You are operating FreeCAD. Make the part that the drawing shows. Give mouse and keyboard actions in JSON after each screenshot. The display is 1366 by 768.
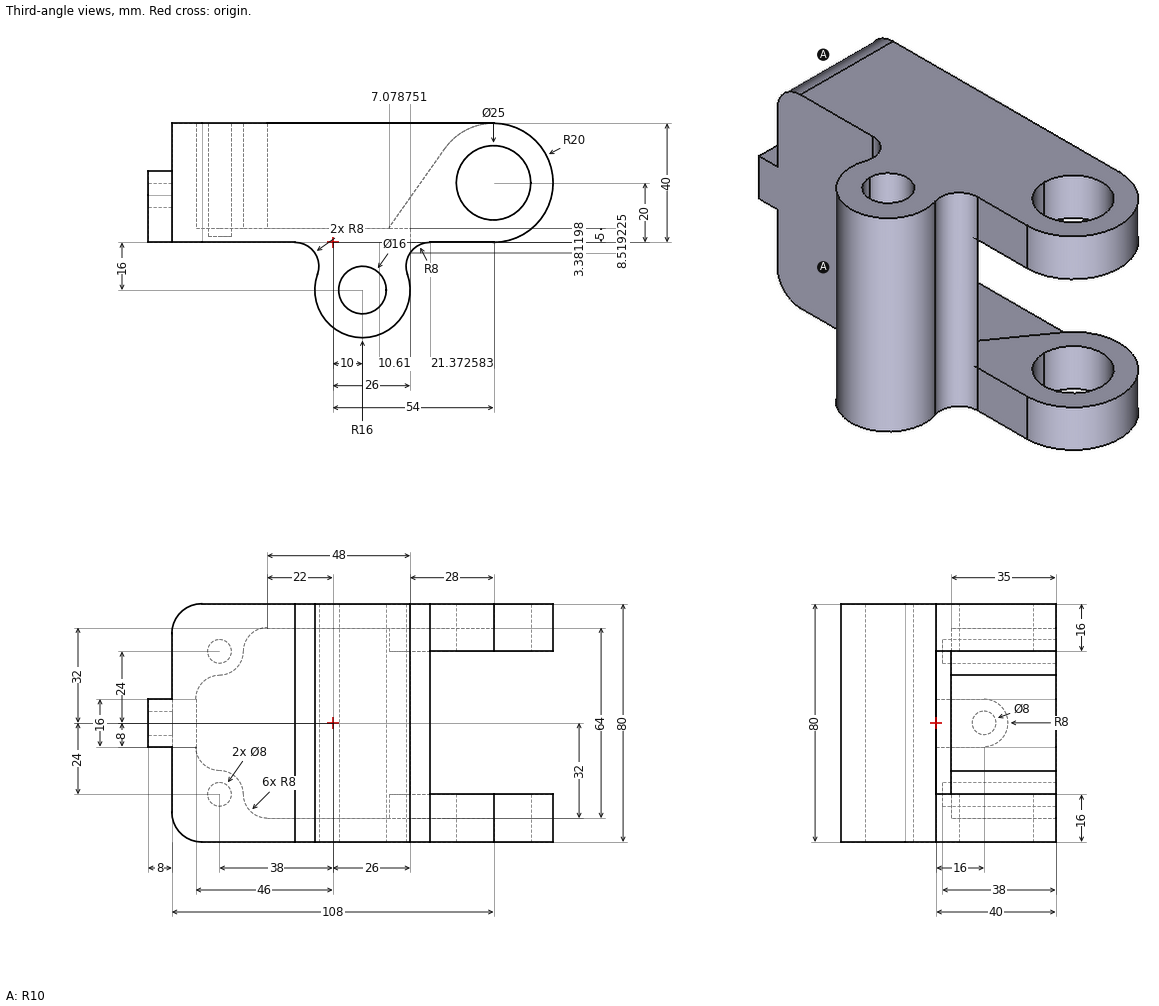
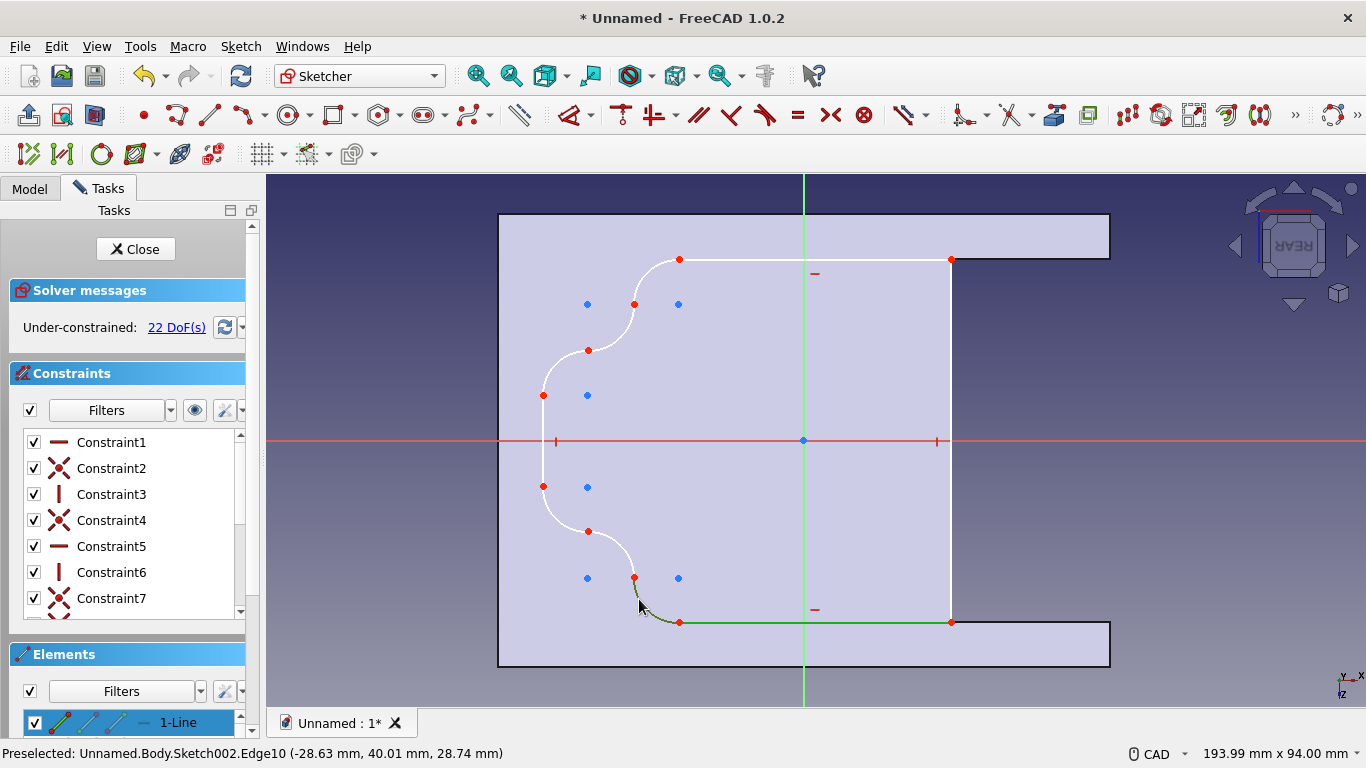
{"action": "key", "text": "t"}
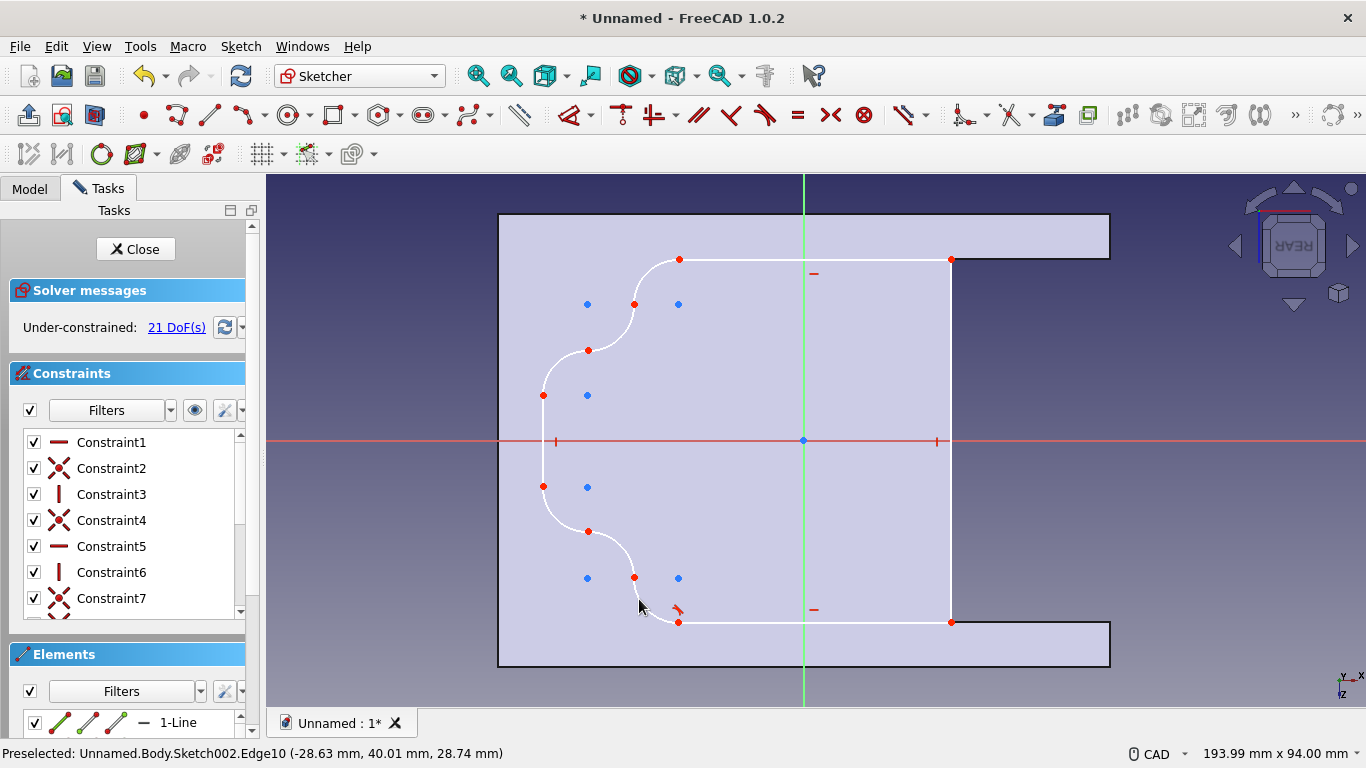
{"action": "left_click", "coordinate": [869, 260]}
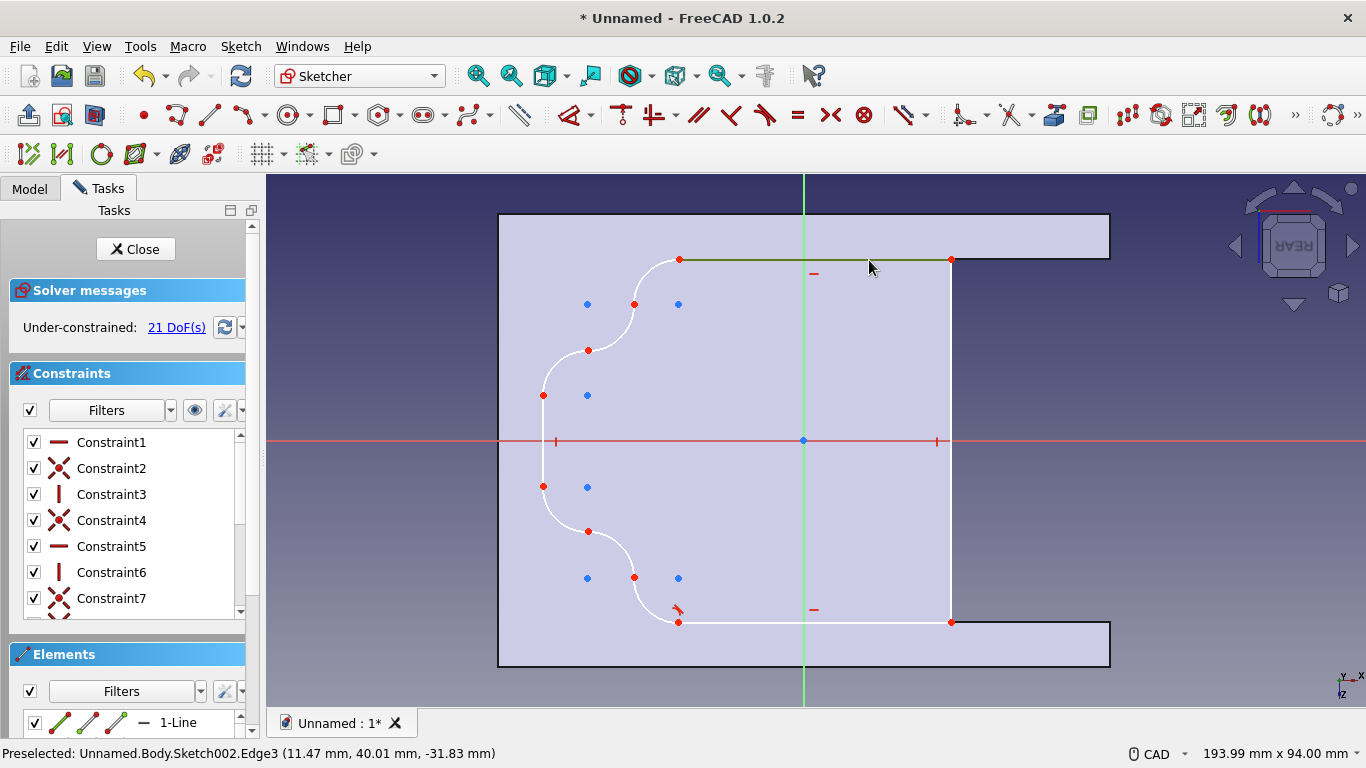
{"action": "left_click", "coordinate": [658, 265]}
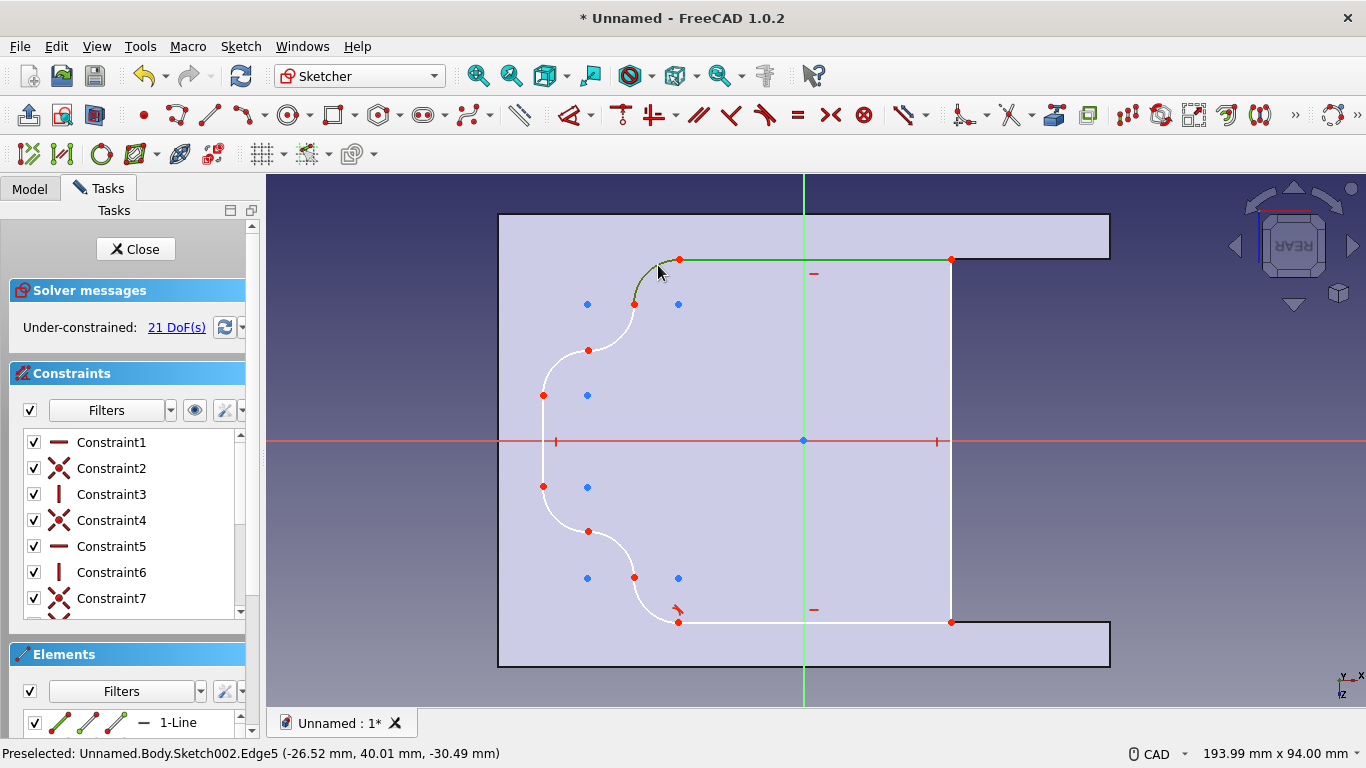
{"action": "key", "text": "t"}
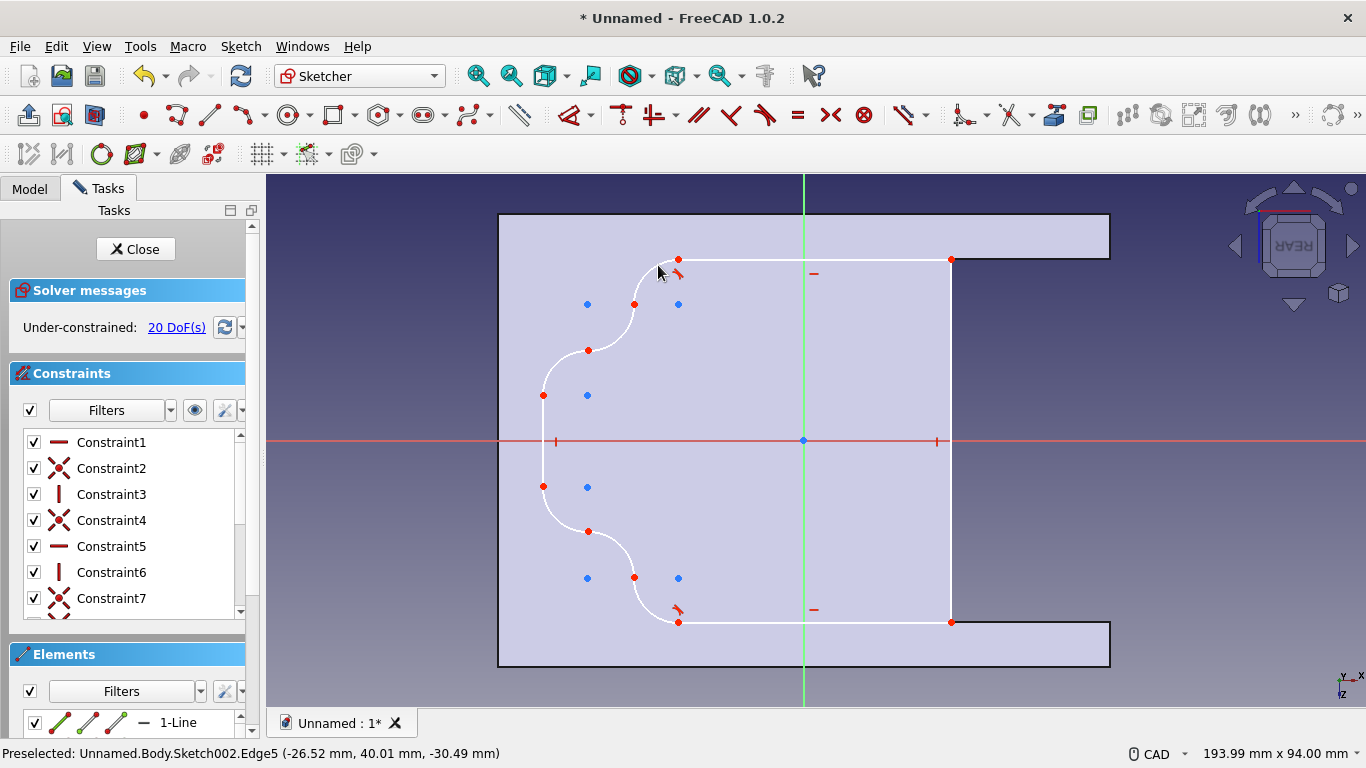
{"action": "left_click", "coordinate": [543, 423]}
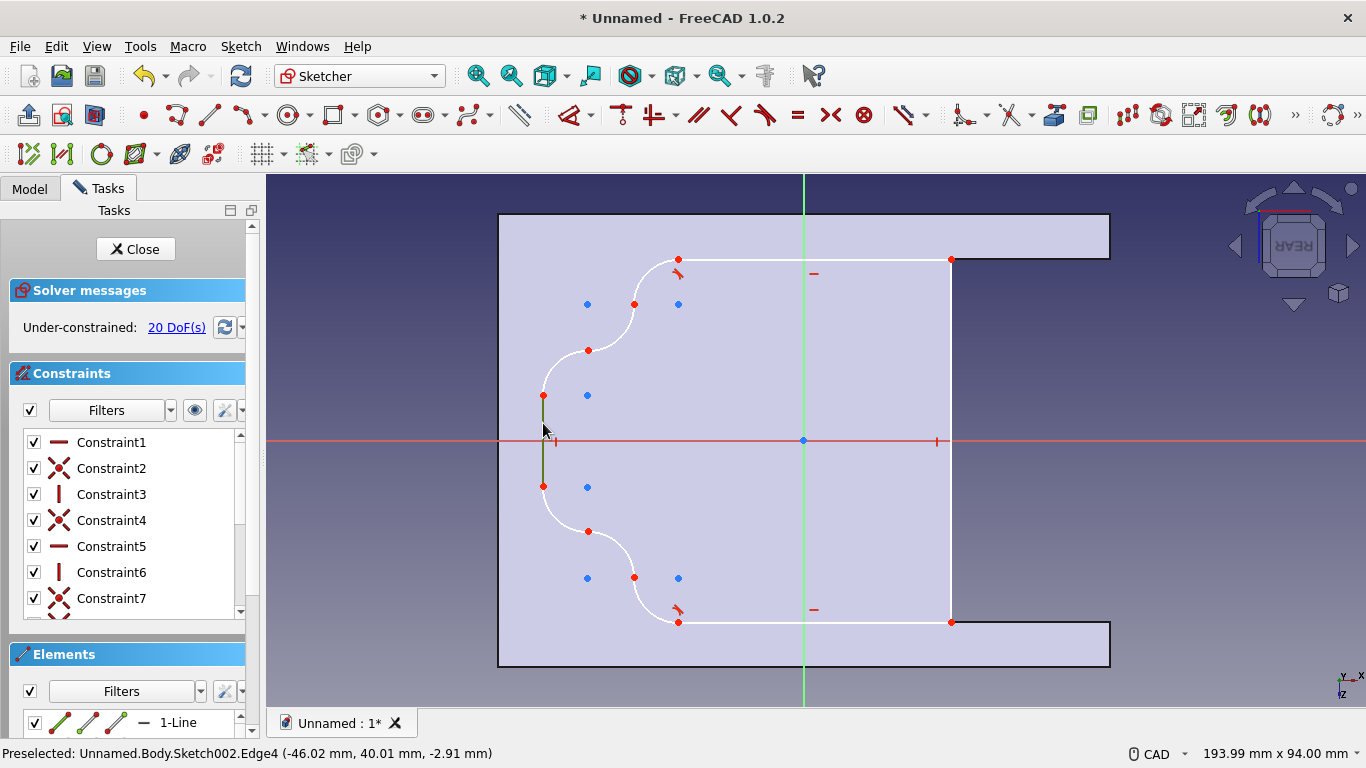
{"action": "left_click", "coordinate": [567, 356]}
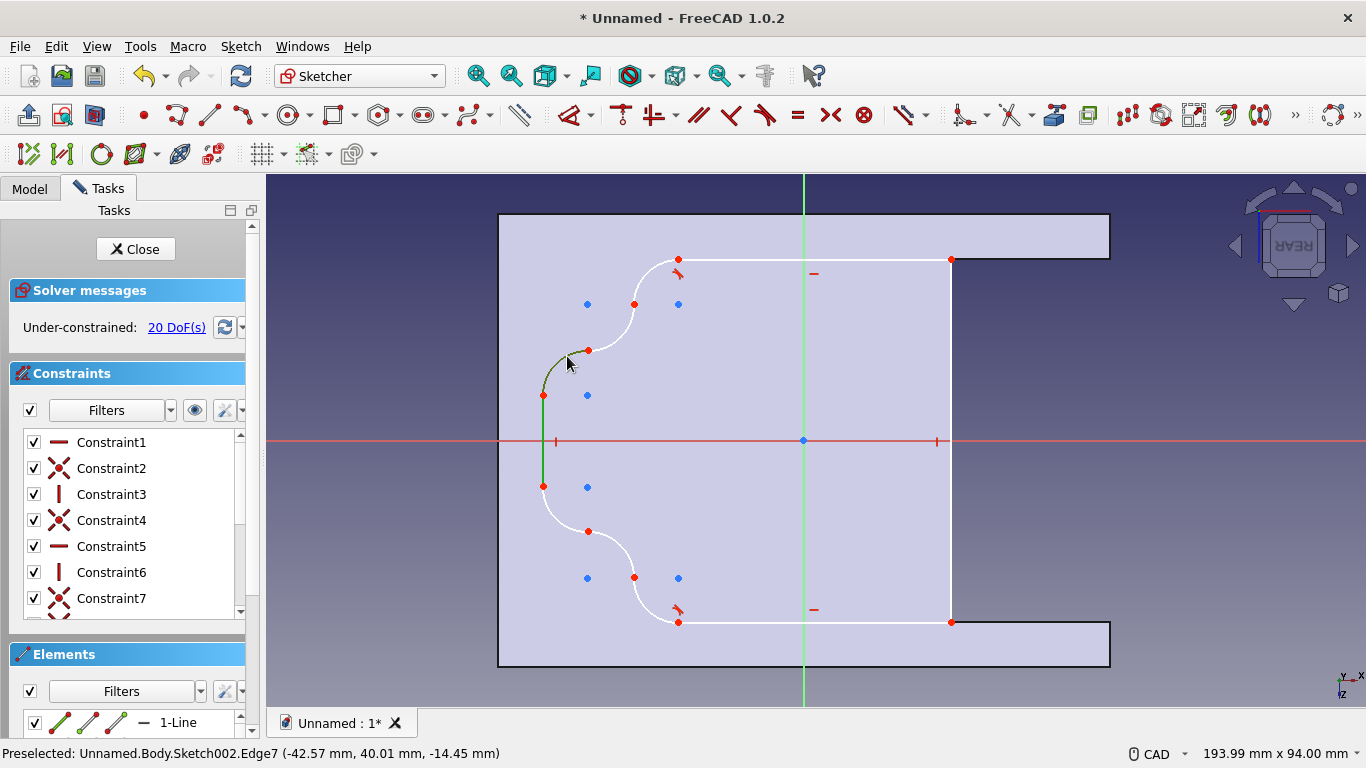
{"action": "key", "text": "t"}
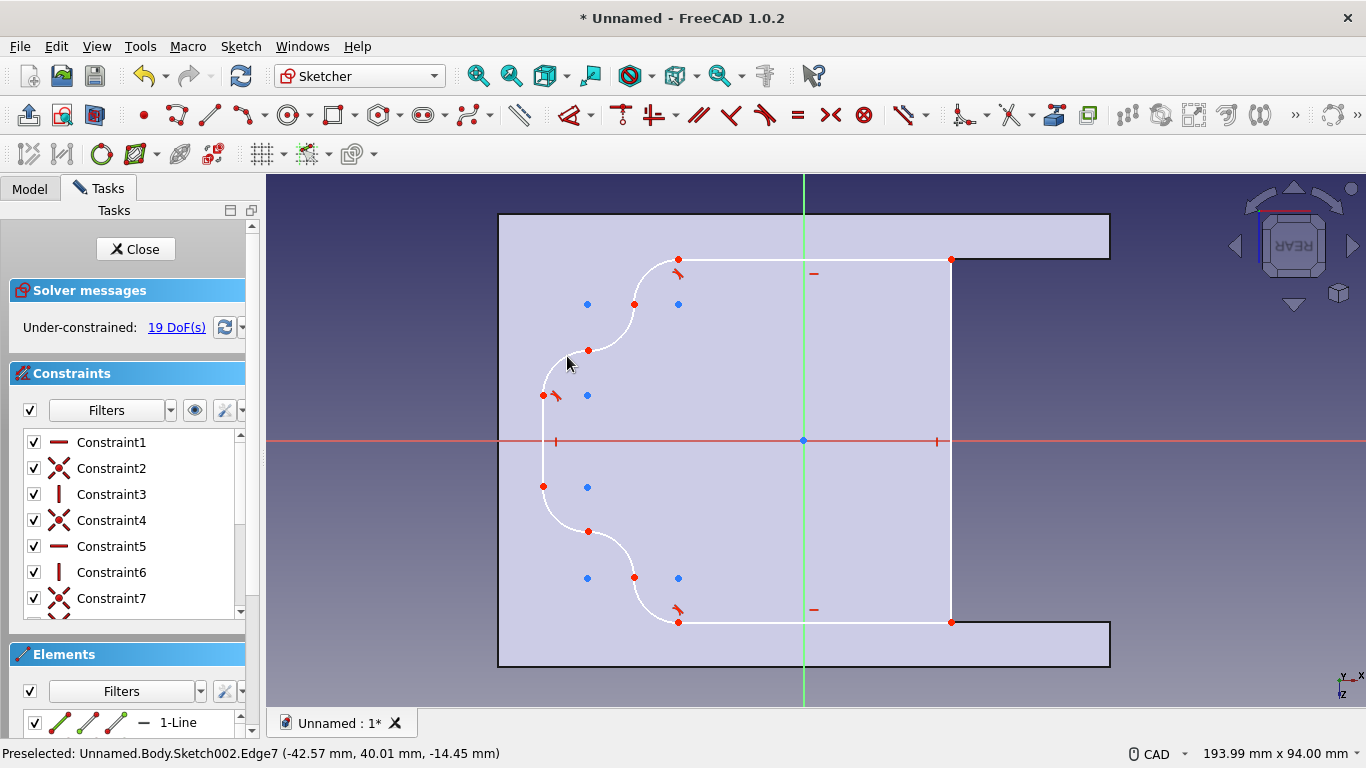
{"action": "left_click", "coordinate": [543, 423]}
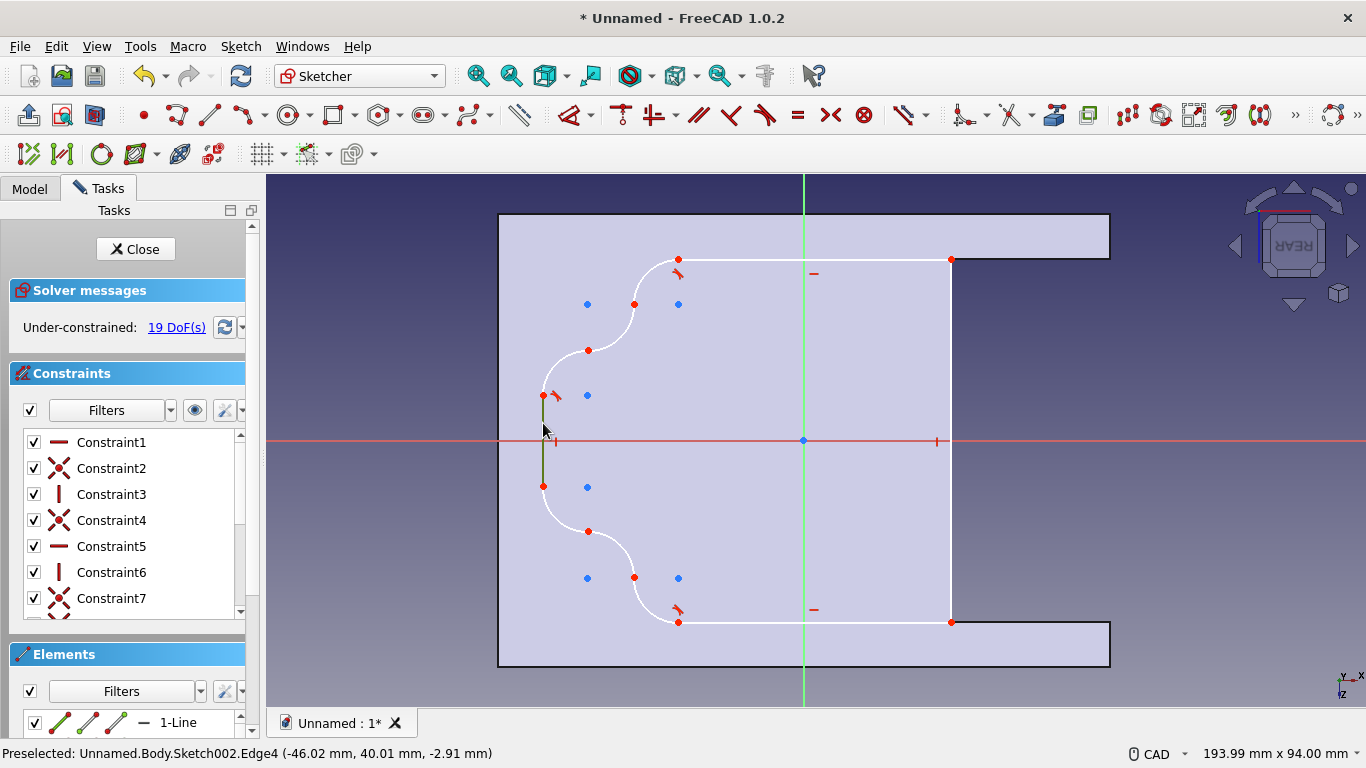
{"action": "left_click", "coordinate": [548, 508]}